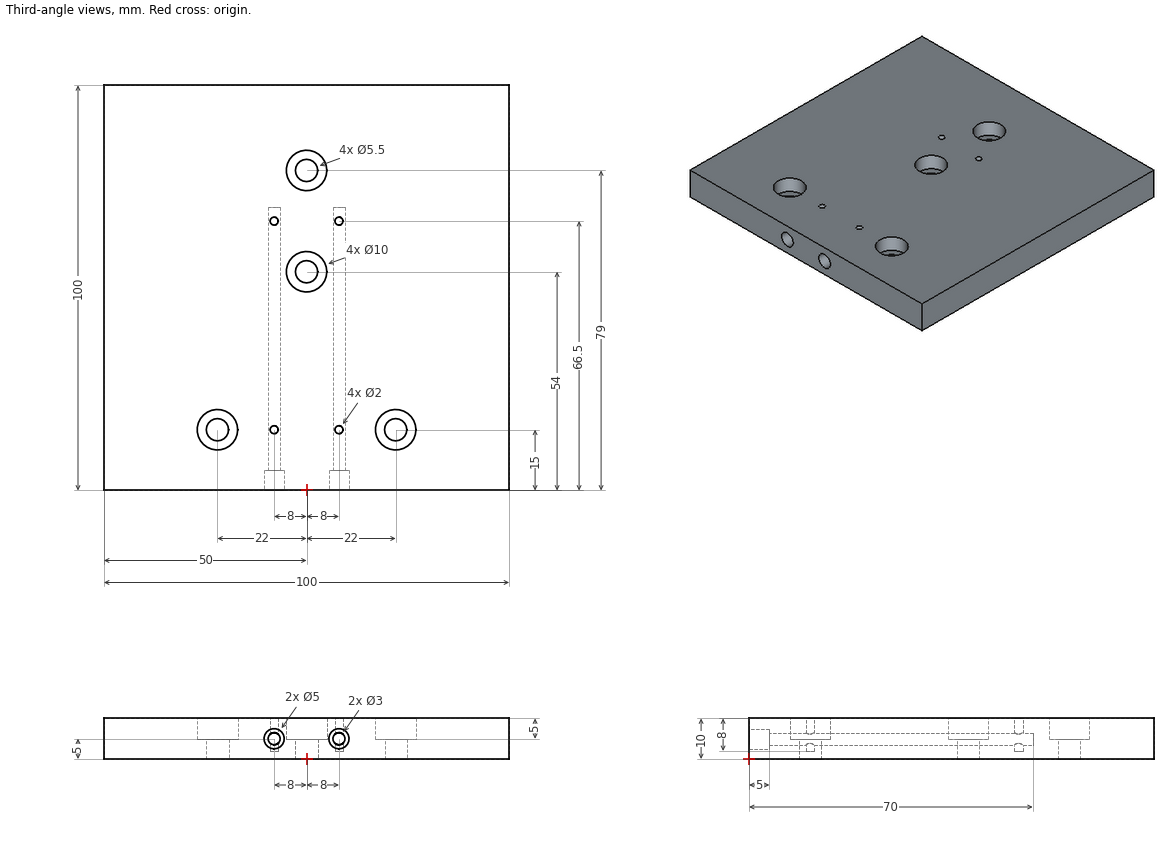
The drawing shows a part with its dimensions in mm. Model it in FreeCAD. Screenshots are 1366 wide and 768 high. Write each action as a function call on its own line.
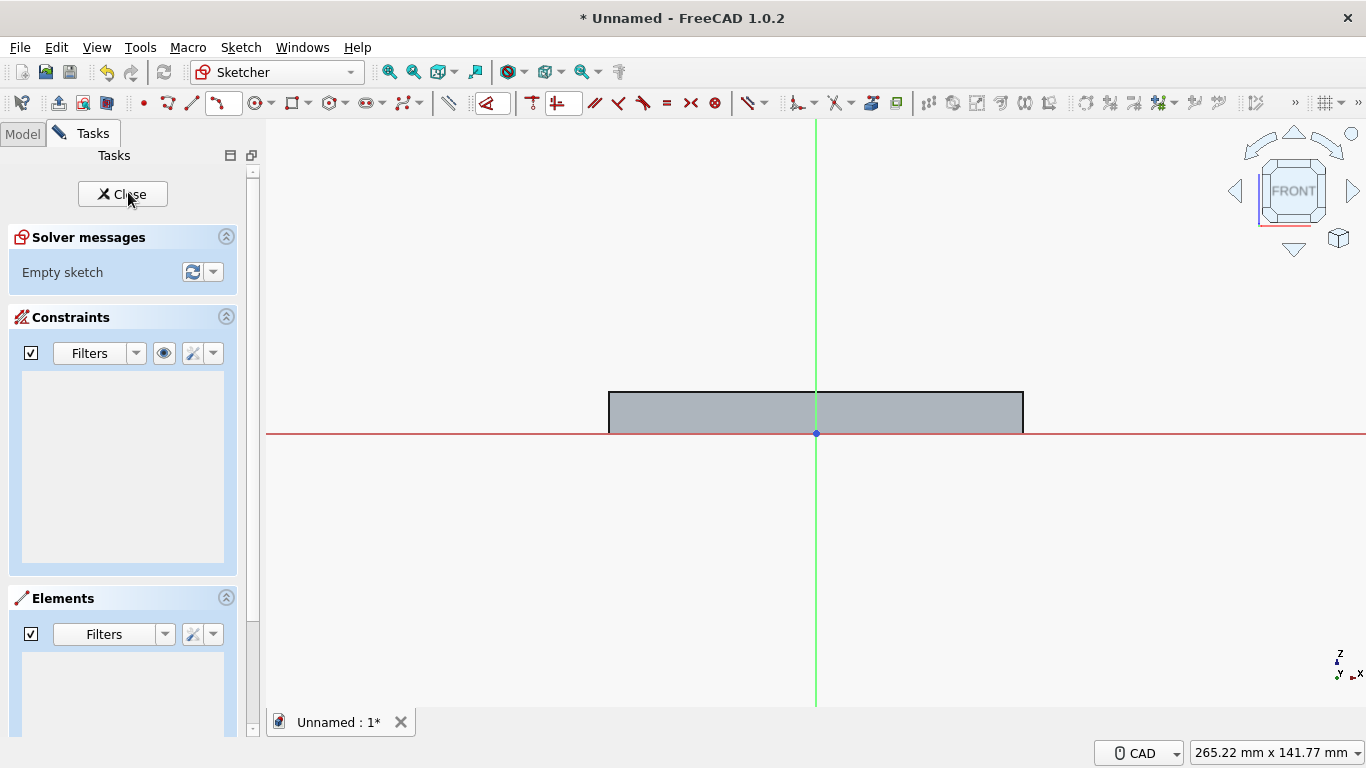
scroll(827, 419, up, 10)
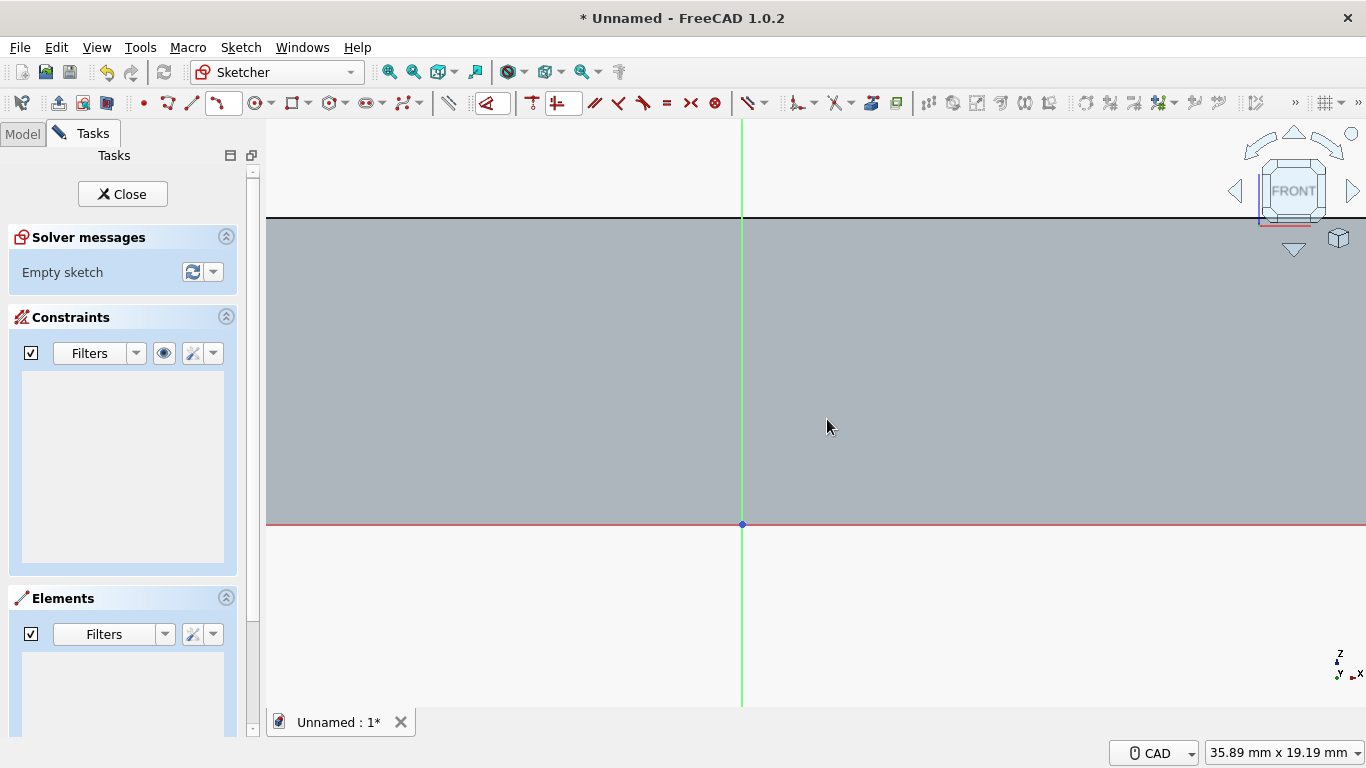
click(256, 104)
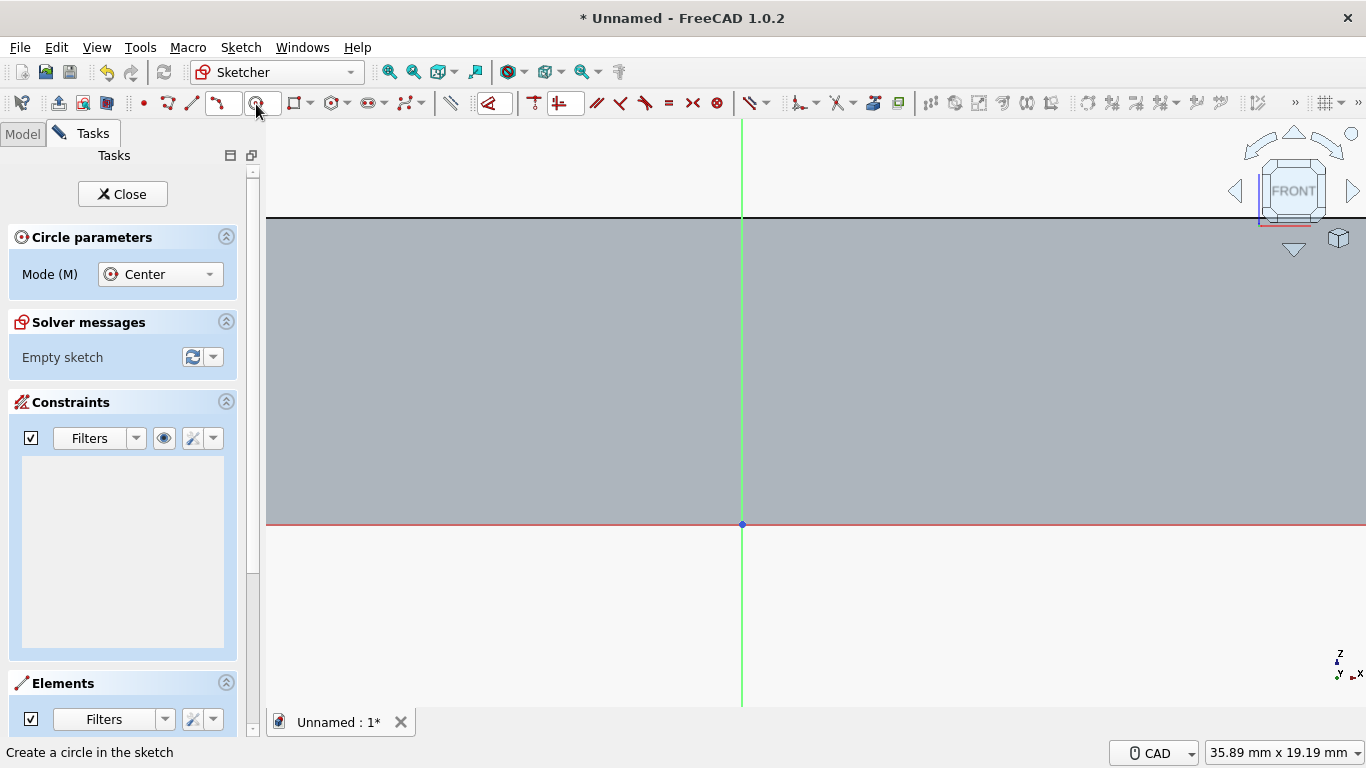
click(497, 371)
click(551, 317)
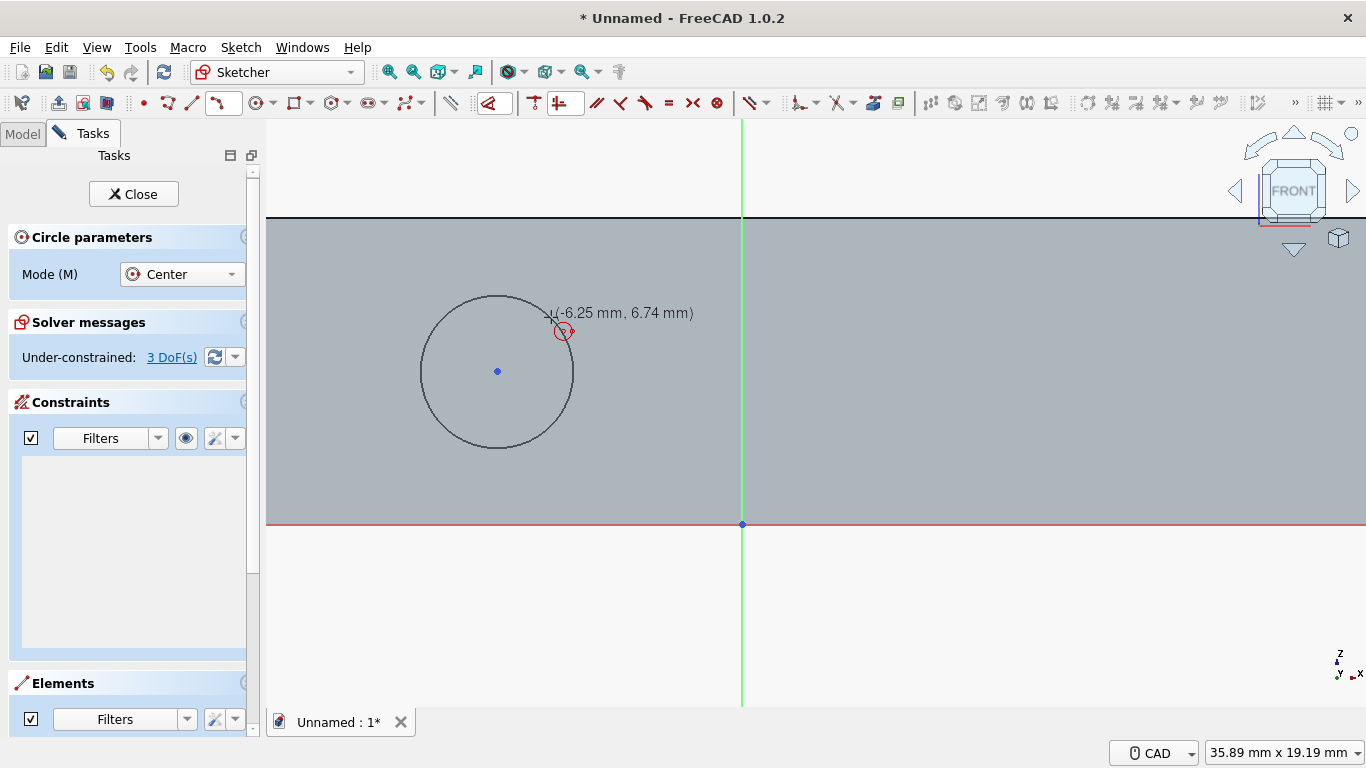
click(988, 371)
click(1042, 317)
key(Escape)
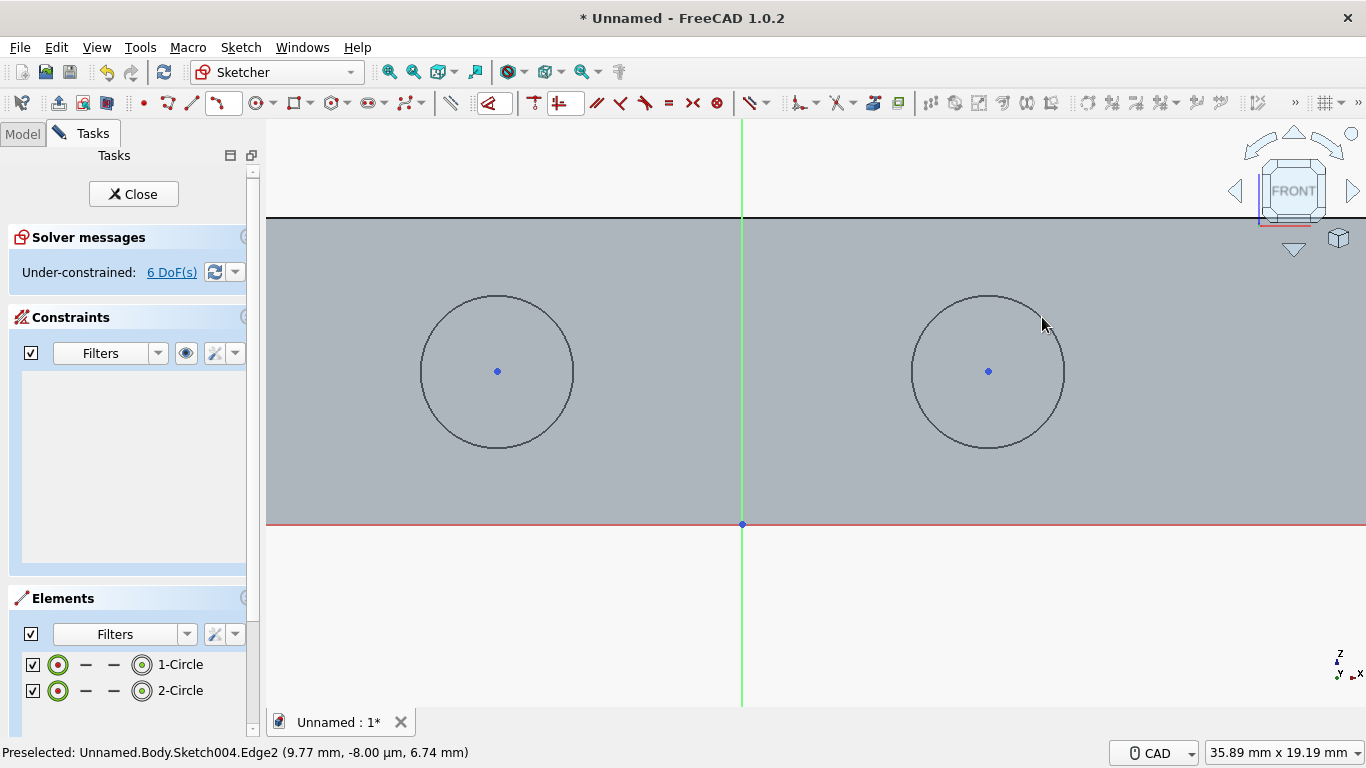
click(551, 318)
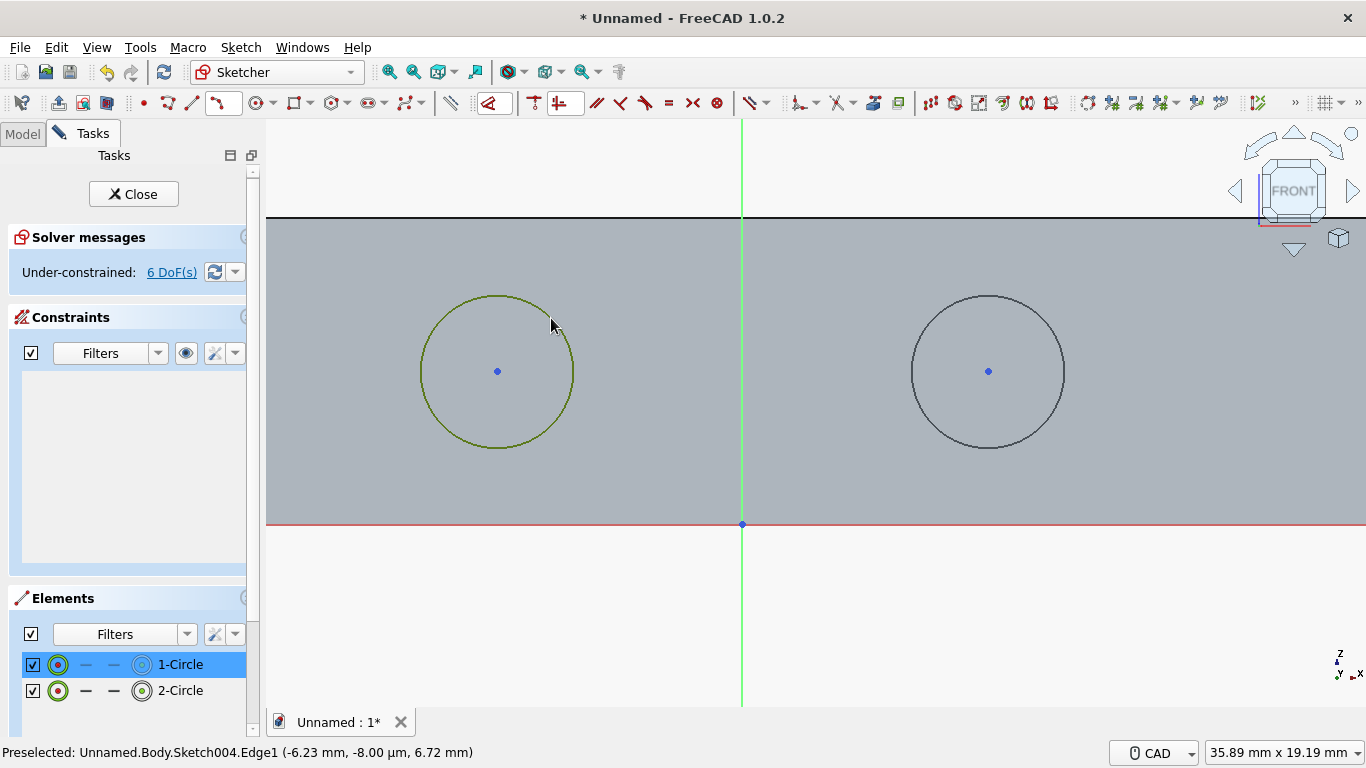
click(1042, 318)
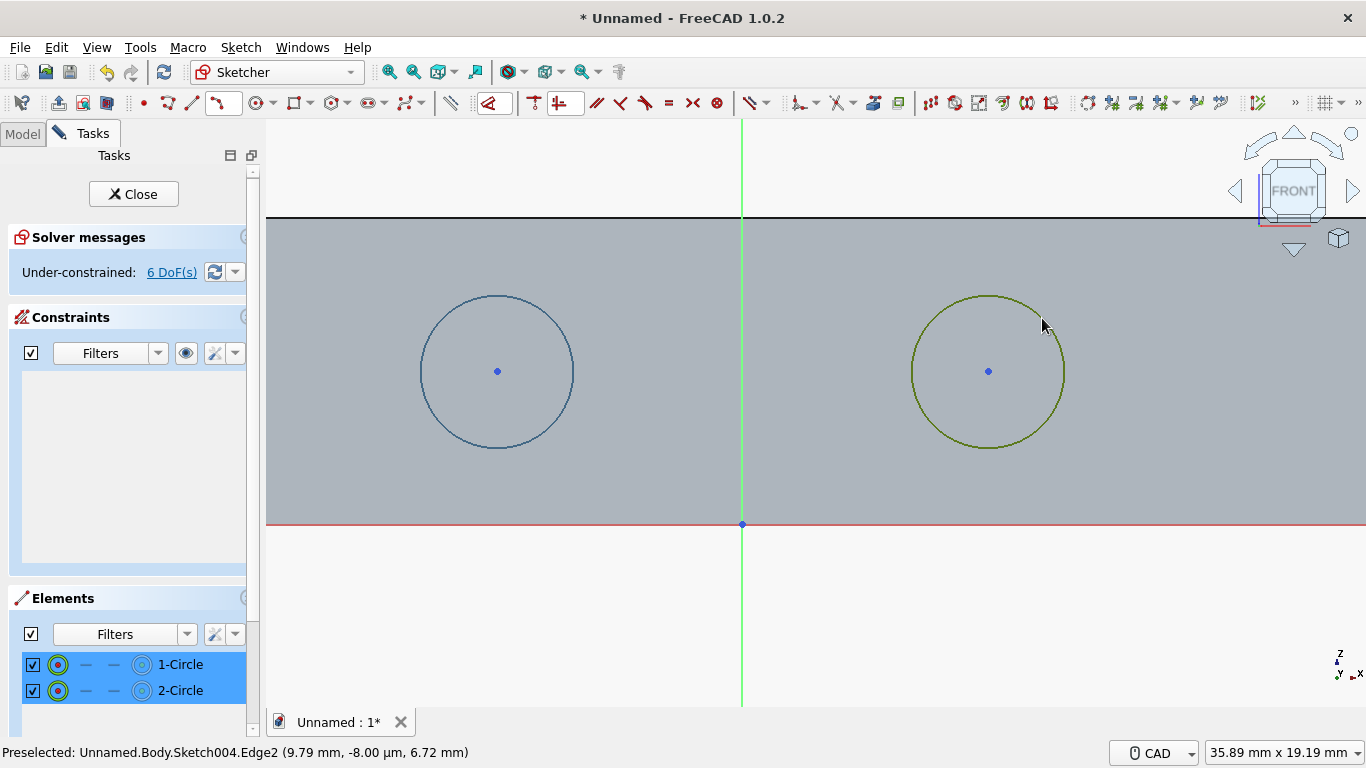
click(670, 104)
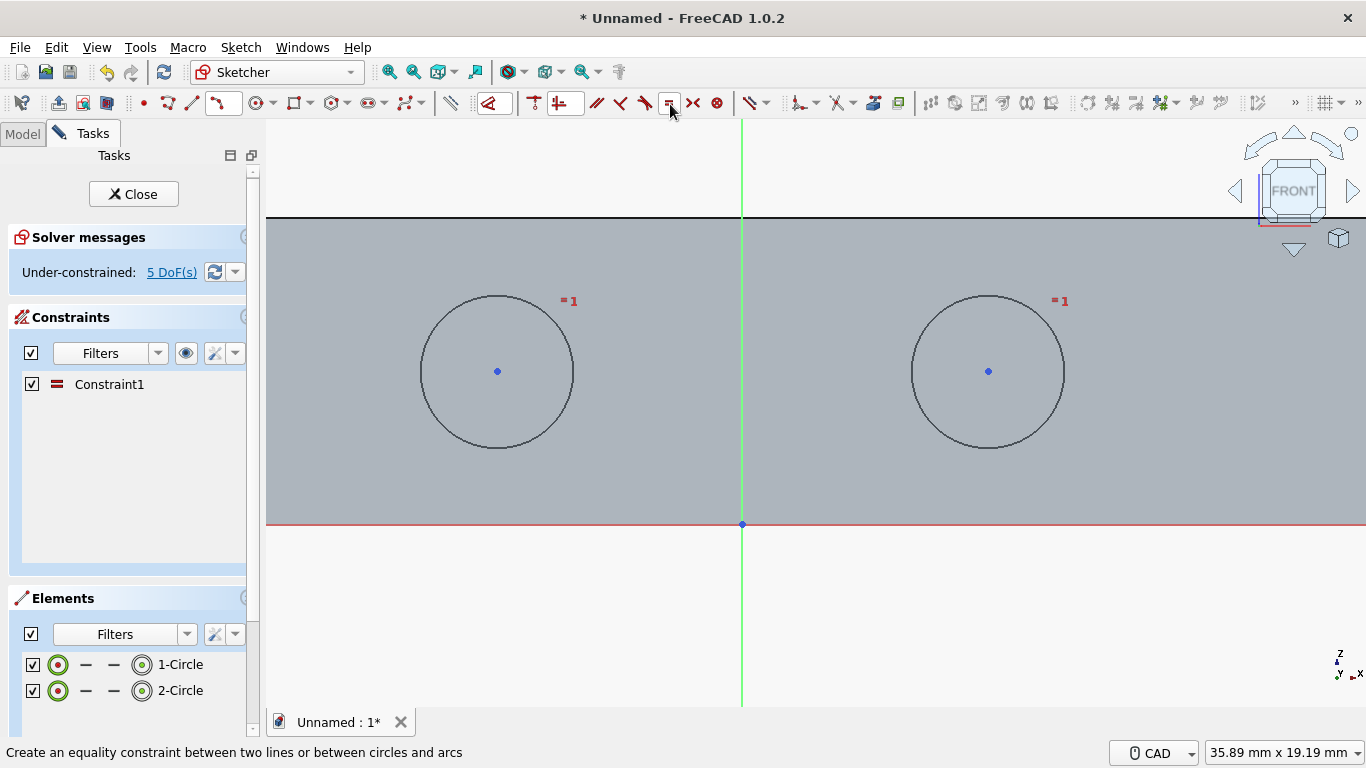
click(551, 318)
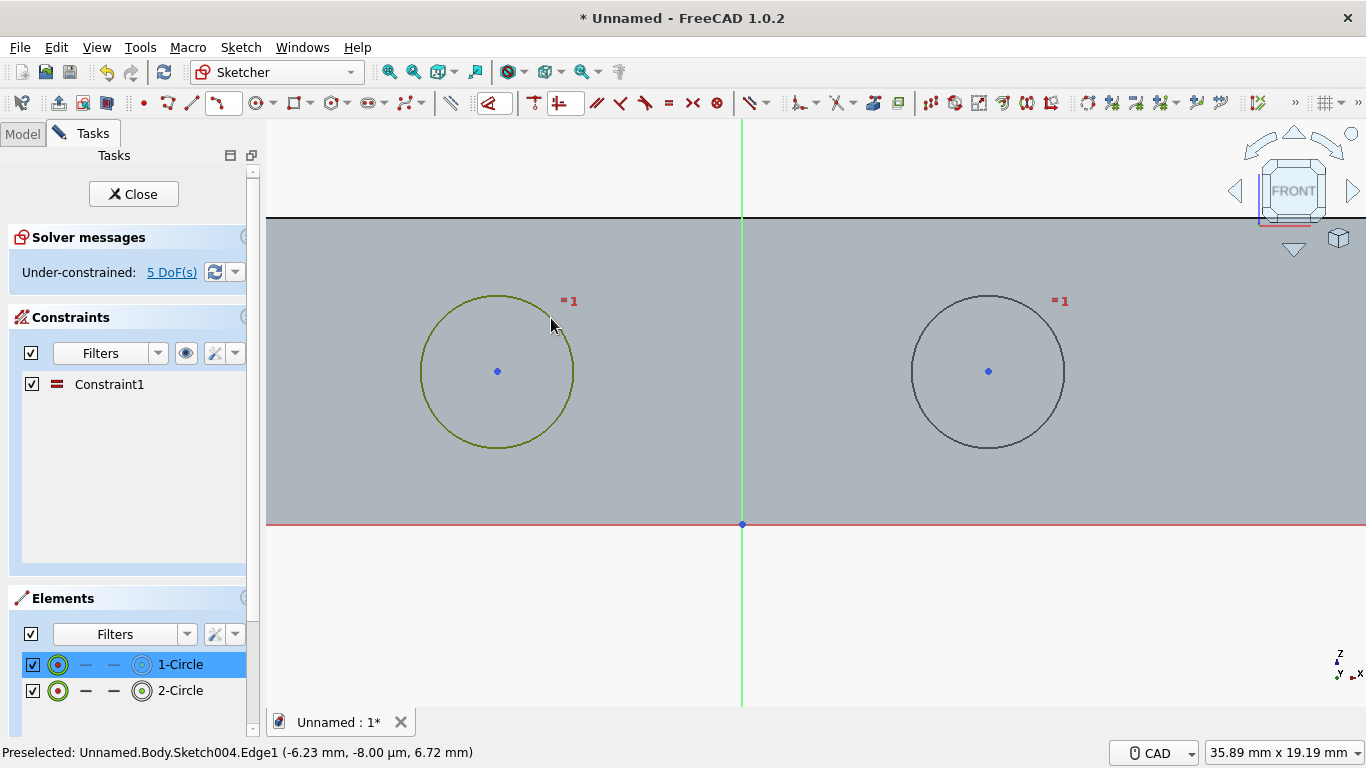
click(506, 104)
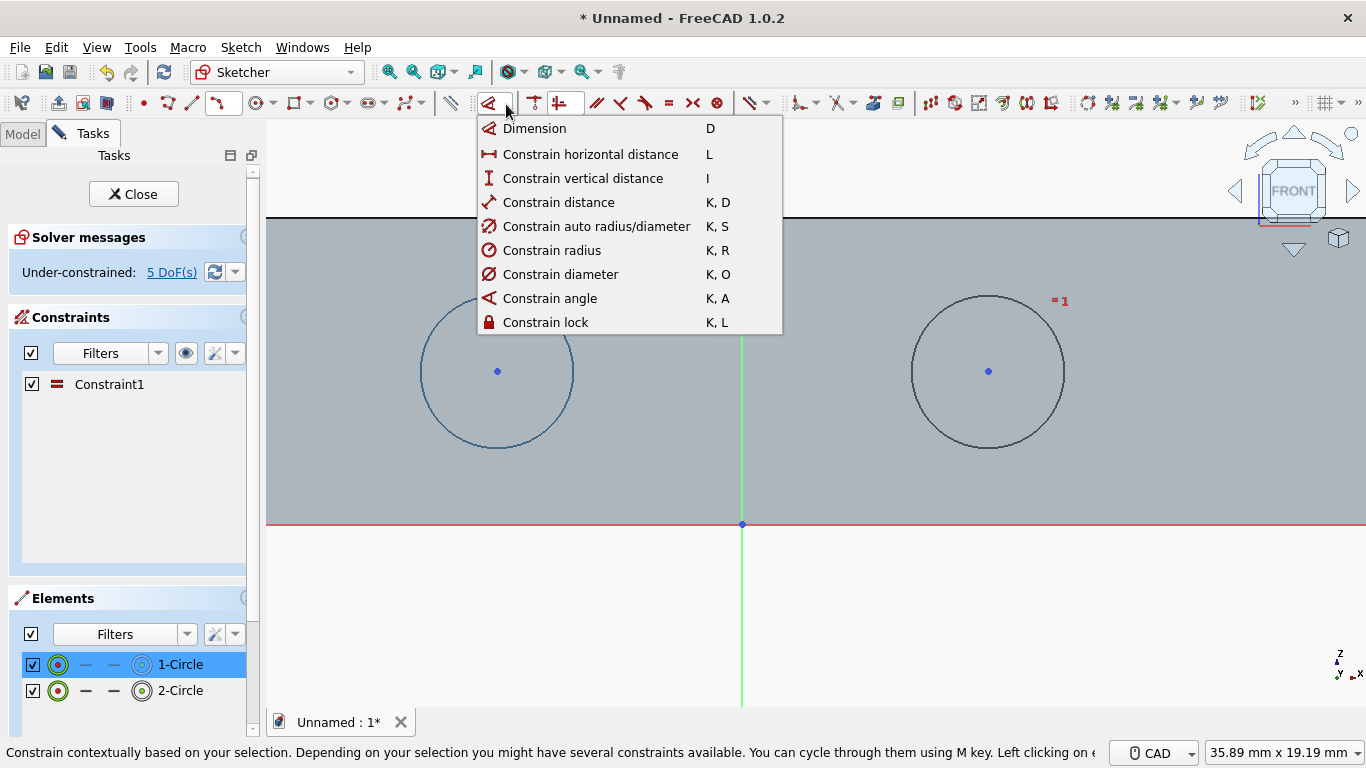
click(630, 274)